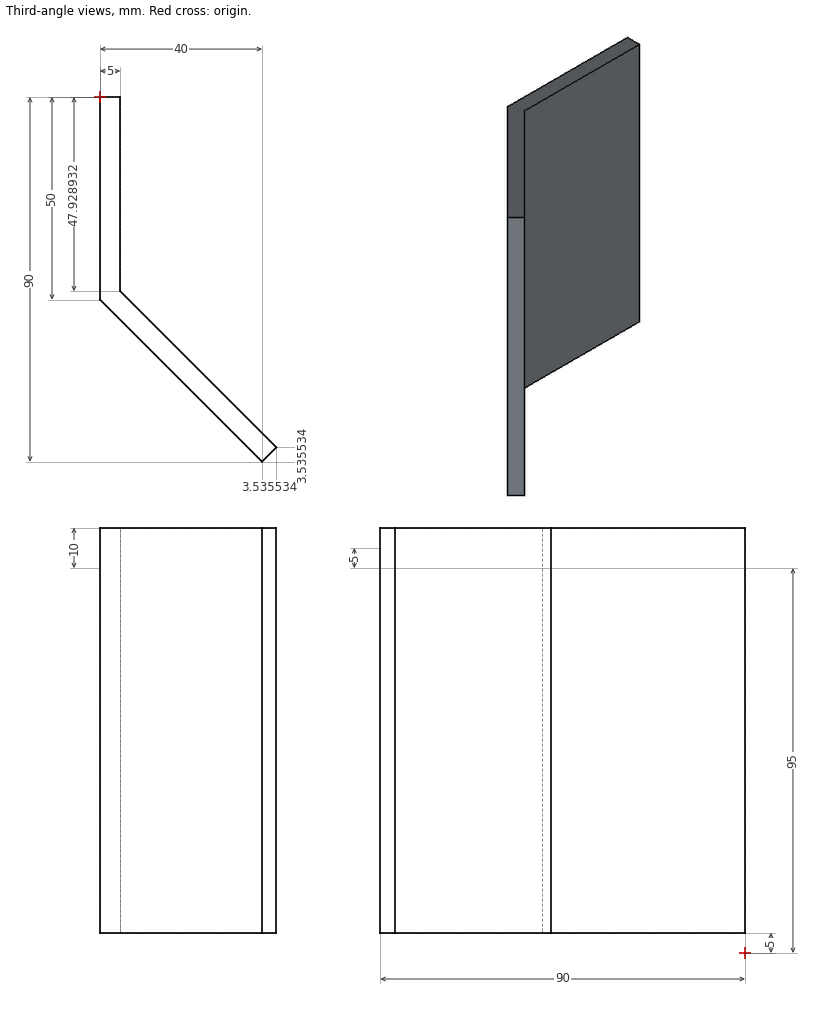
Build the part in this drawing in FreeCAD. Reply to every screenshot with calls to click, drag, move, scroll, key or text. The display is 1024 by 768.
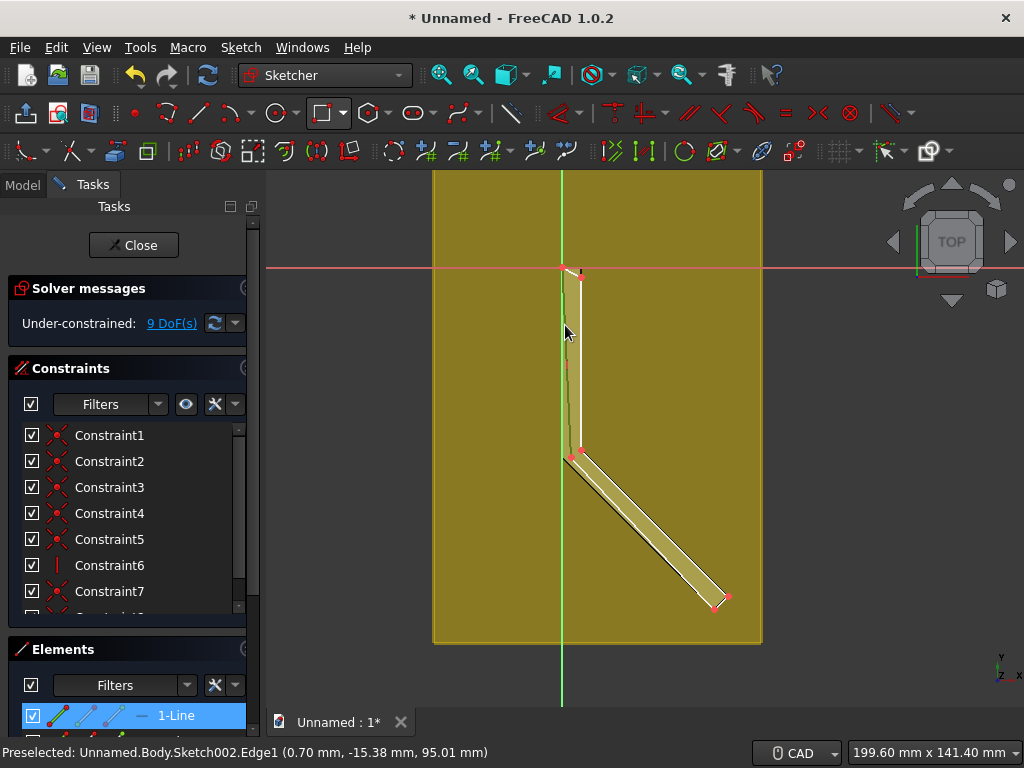
click(668, 114)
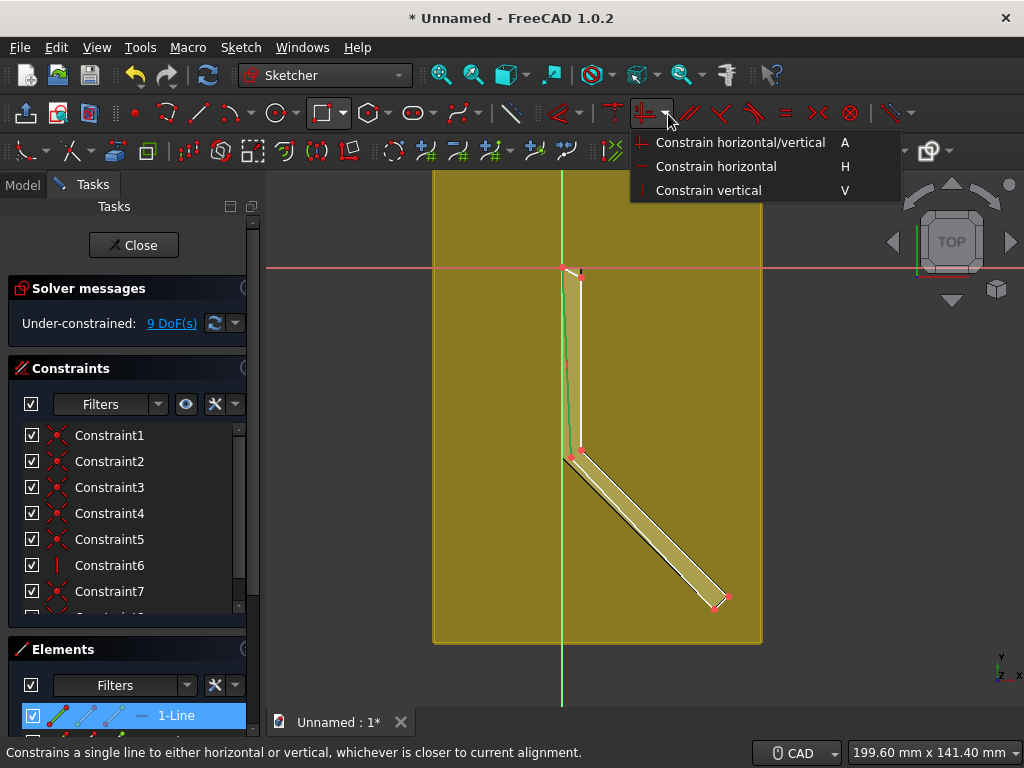
click(766, 190)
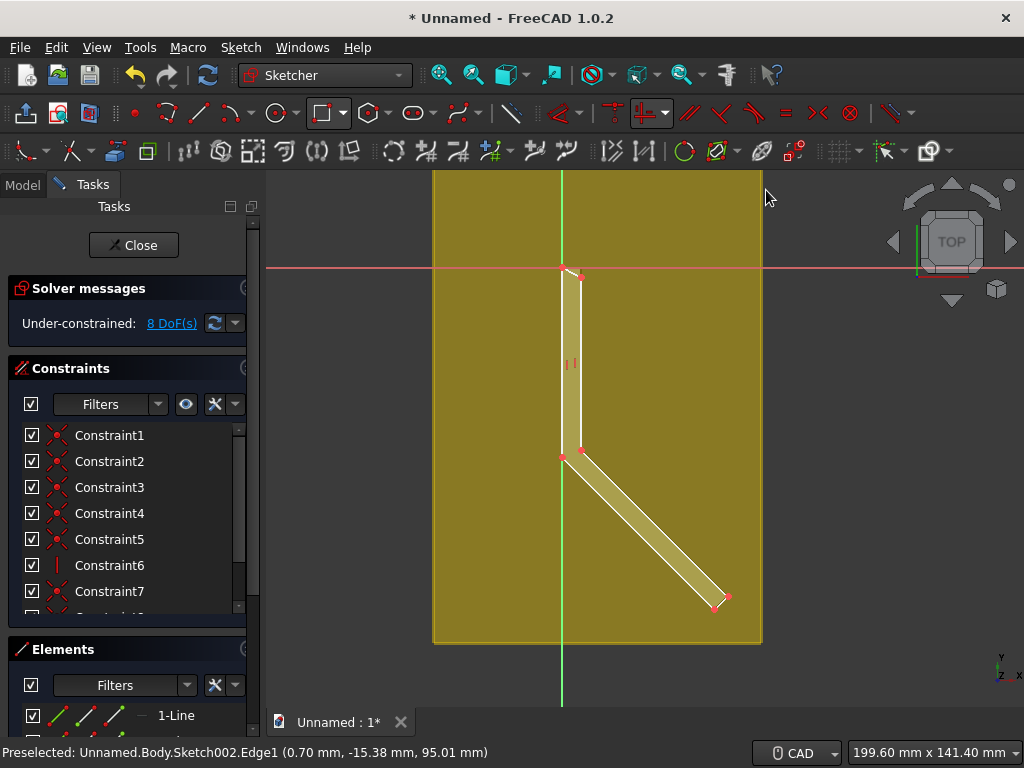
scroll(575, 275, up, 4)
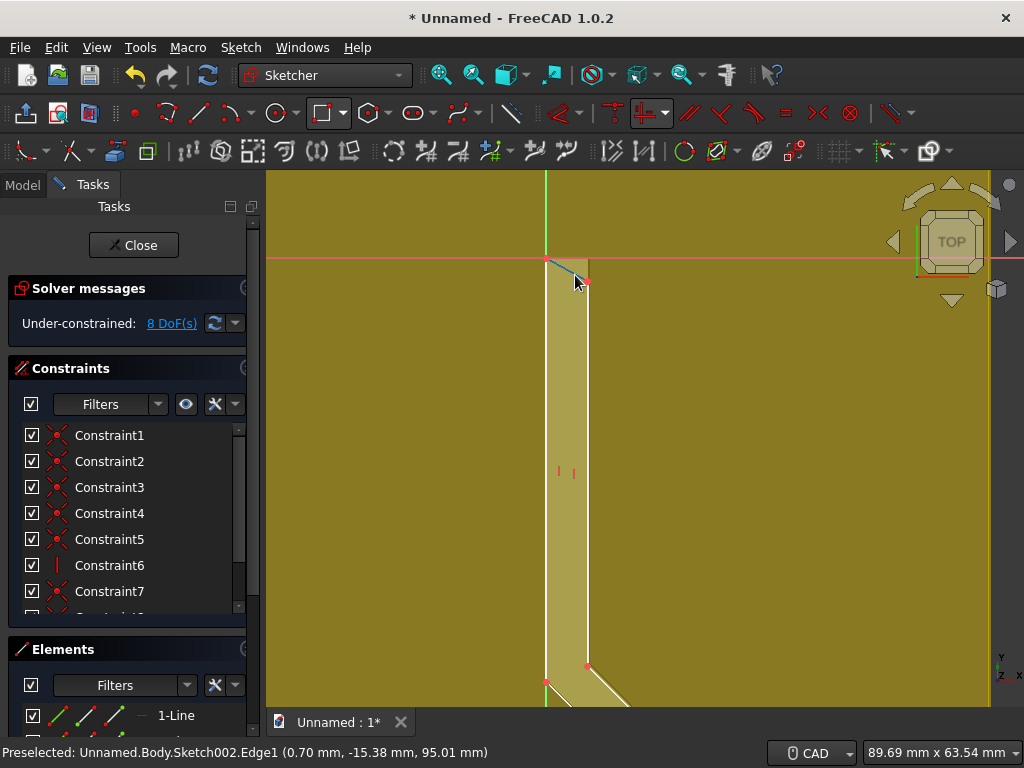
click(575, 274)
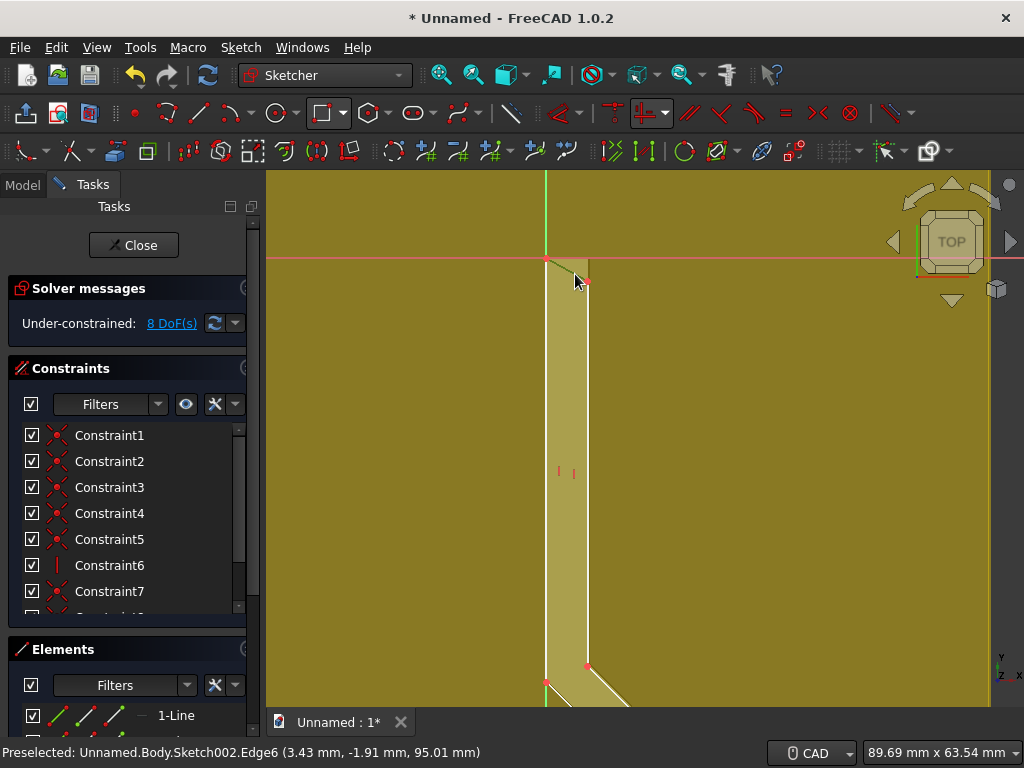
click(668, 114)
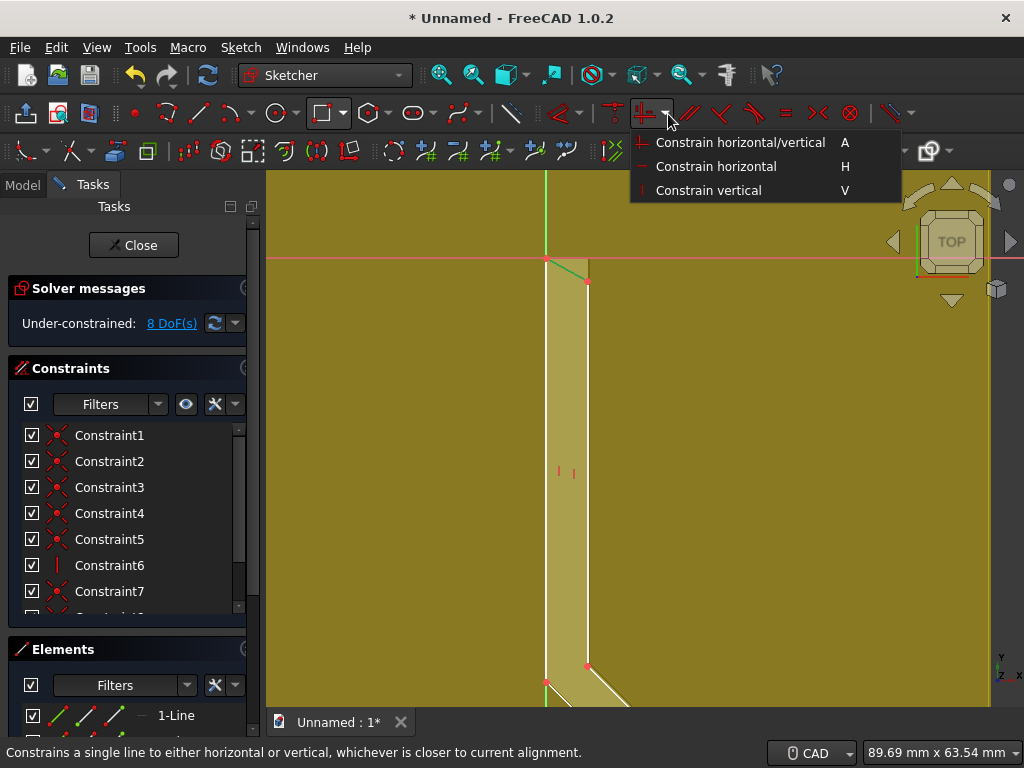
click(766, 166)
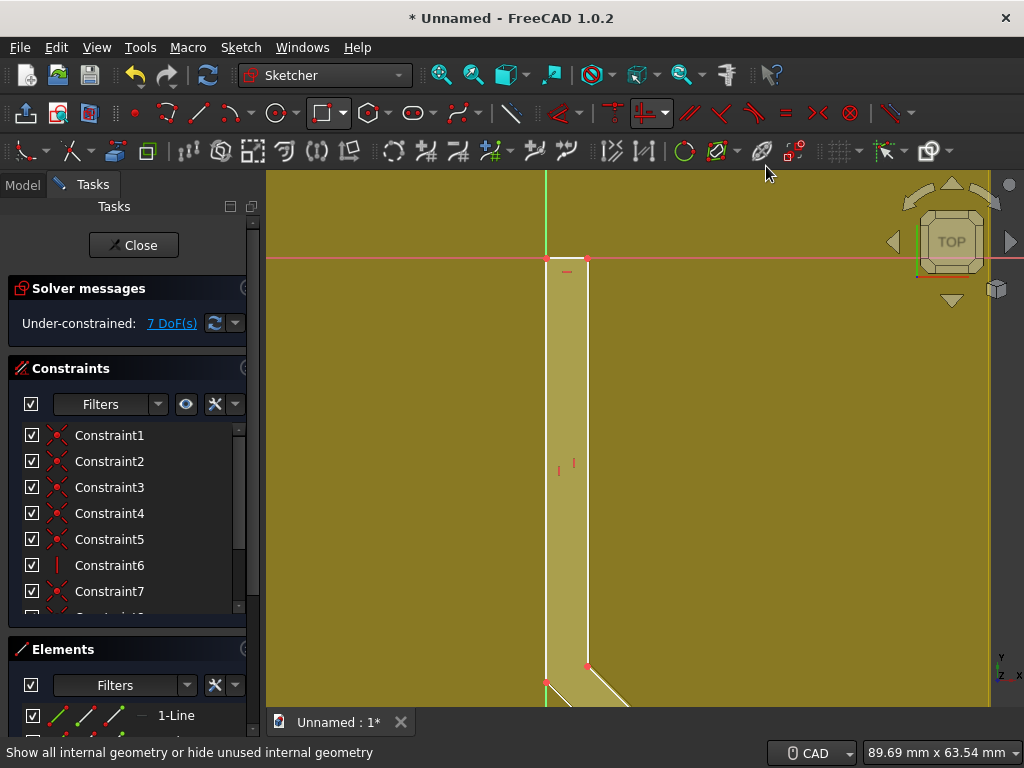
click(558, 114)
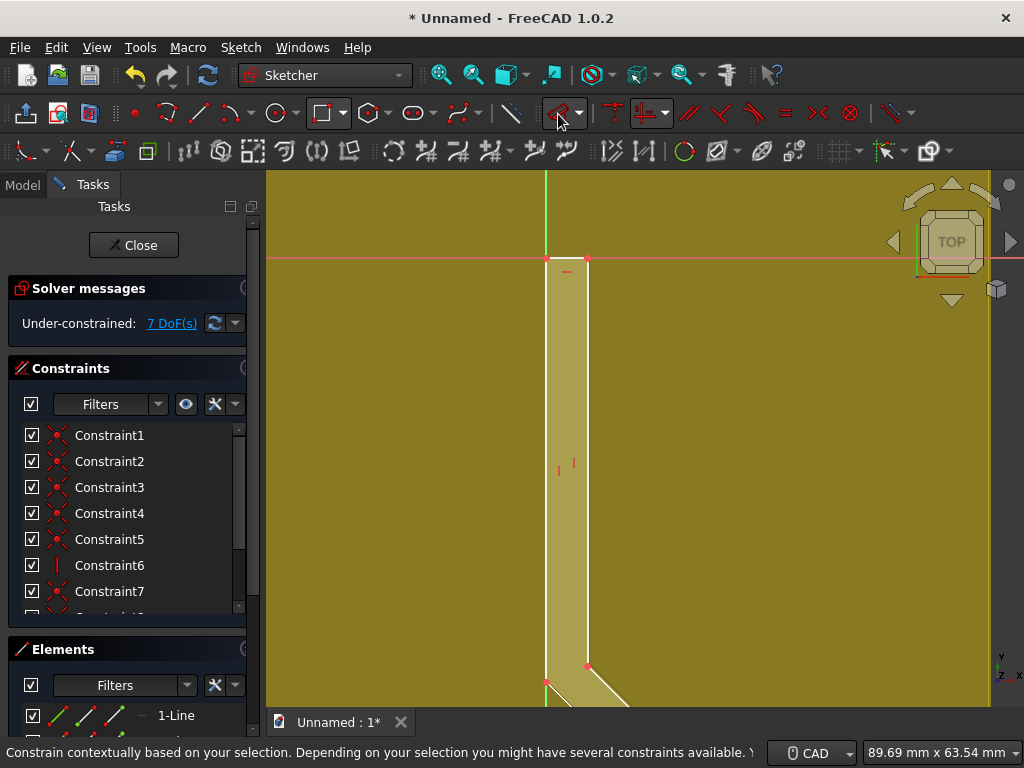
click(575, 258)
click(567, 224)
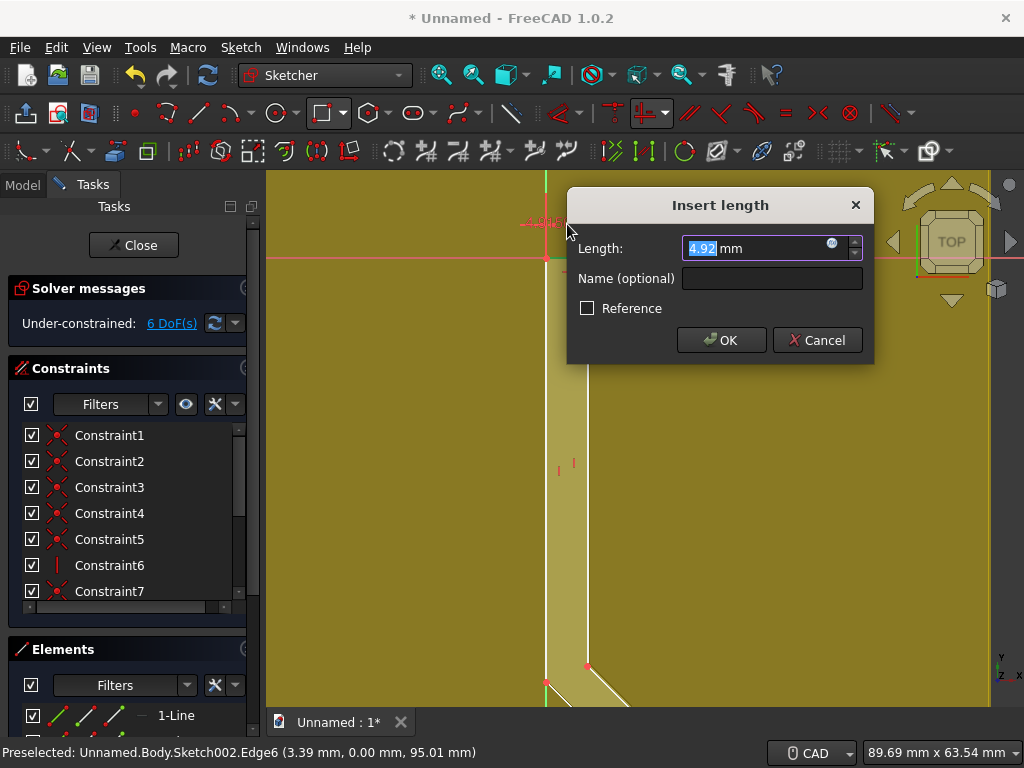
text(5)
key(Return)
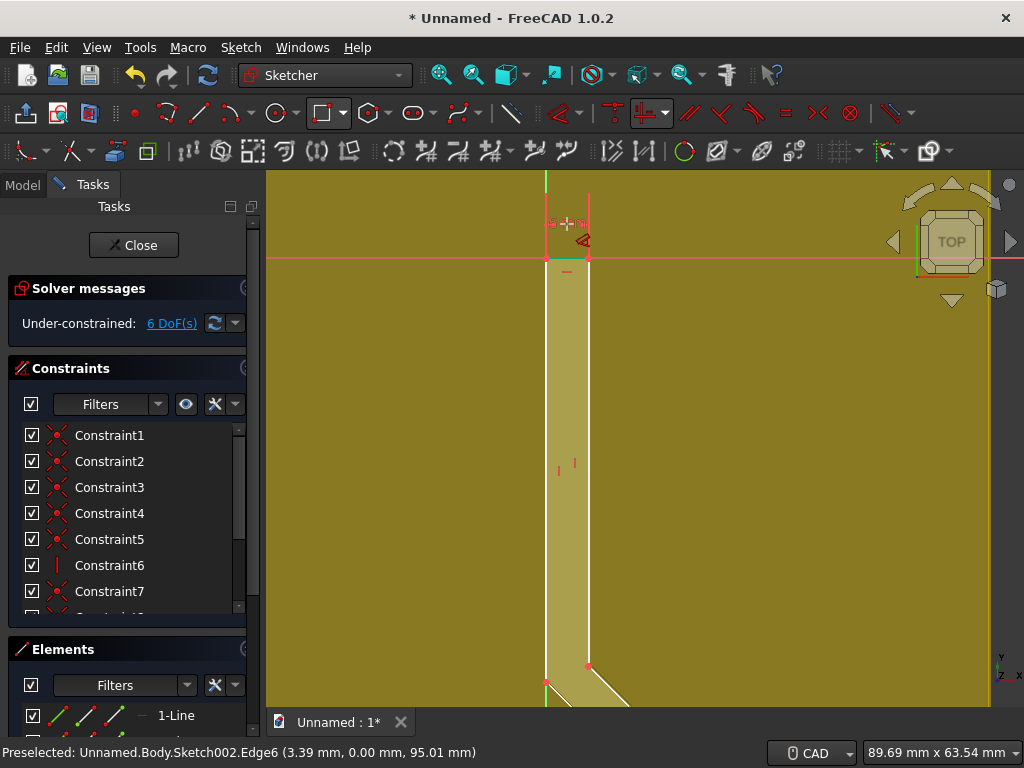
click(546, 385)
click(512, 469)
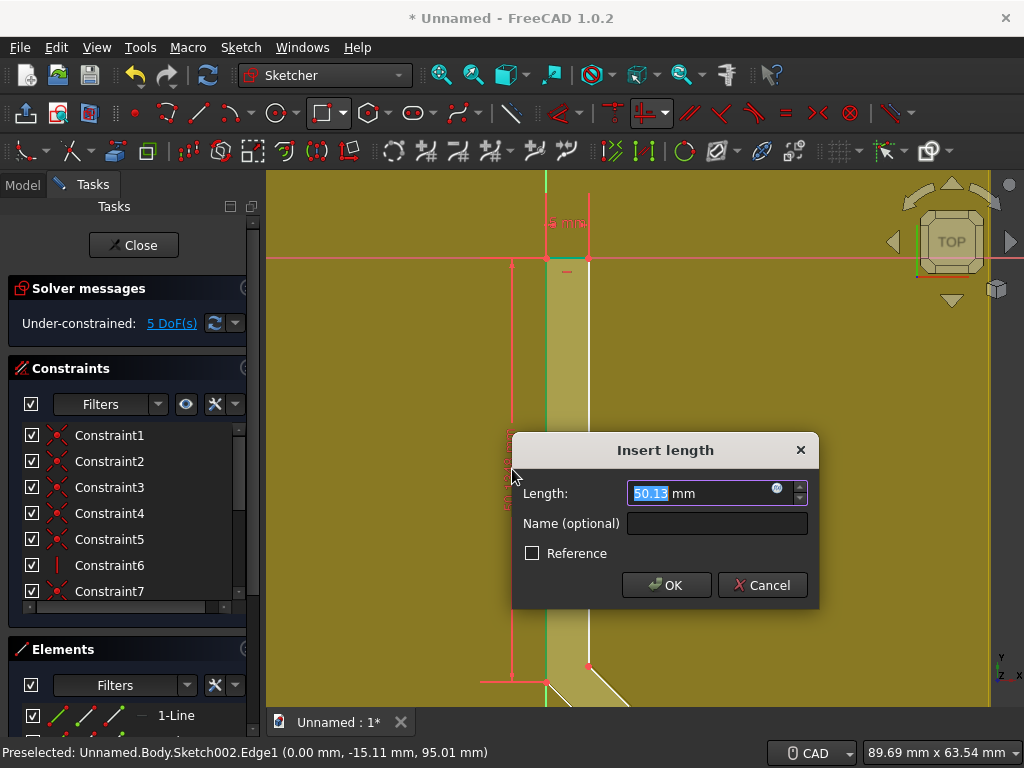
text(50)
key(Return)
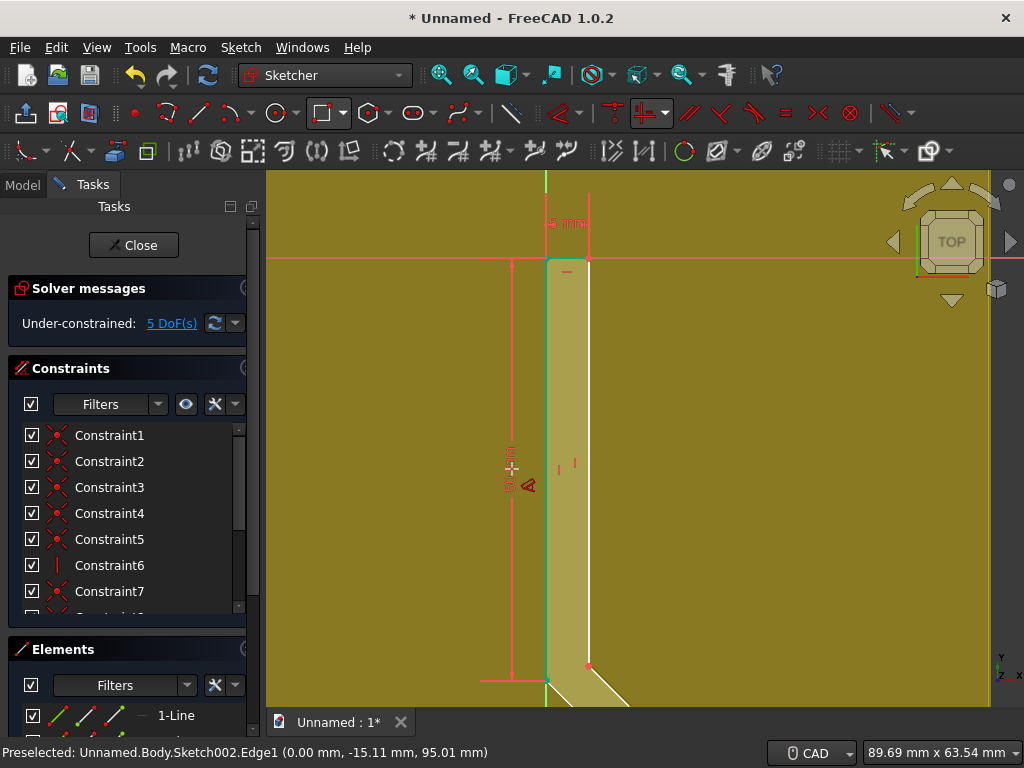
scroll(451, 275, down, 4)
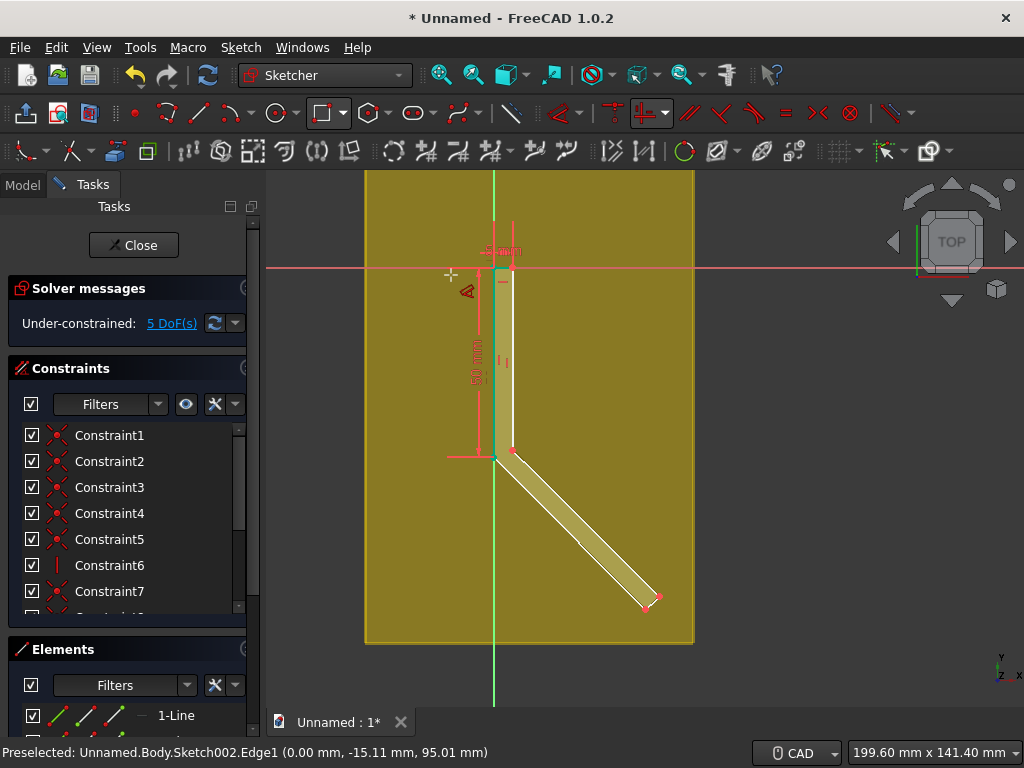
click(646, 610)
click(570, 644)